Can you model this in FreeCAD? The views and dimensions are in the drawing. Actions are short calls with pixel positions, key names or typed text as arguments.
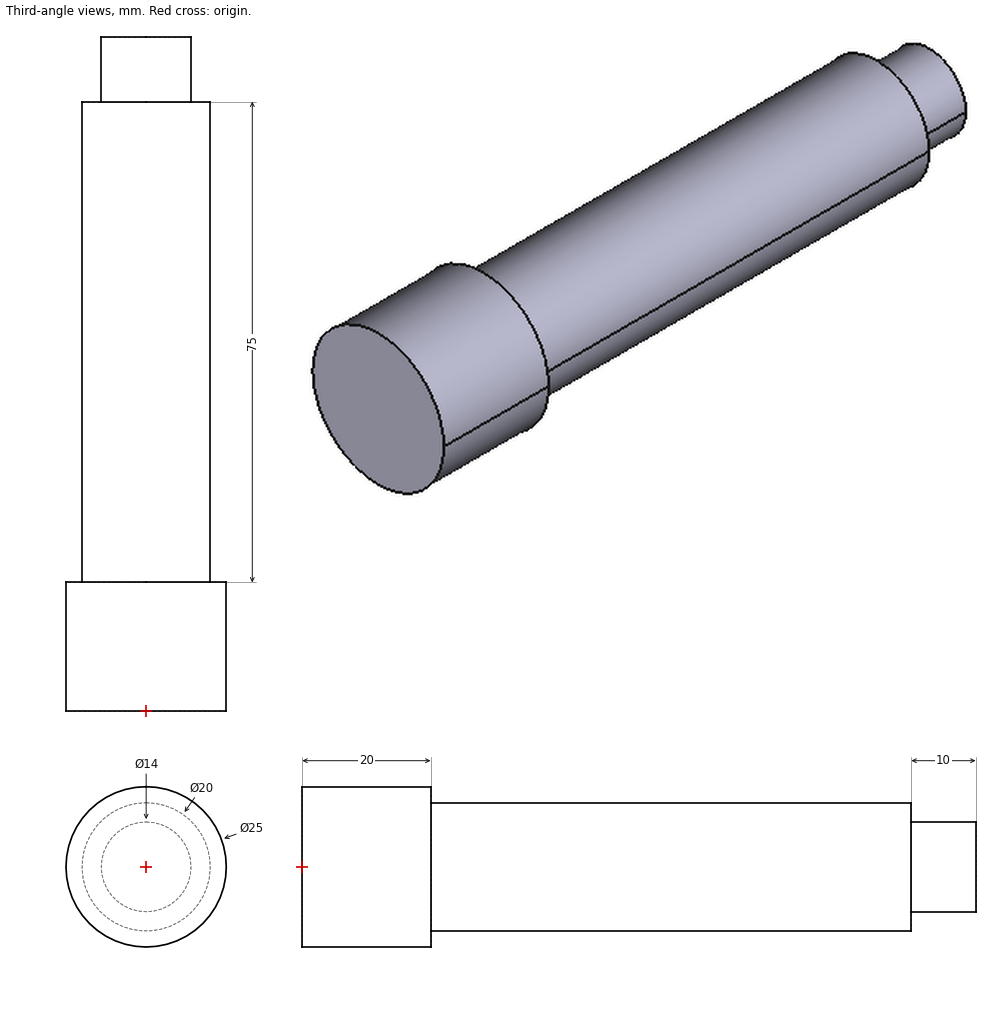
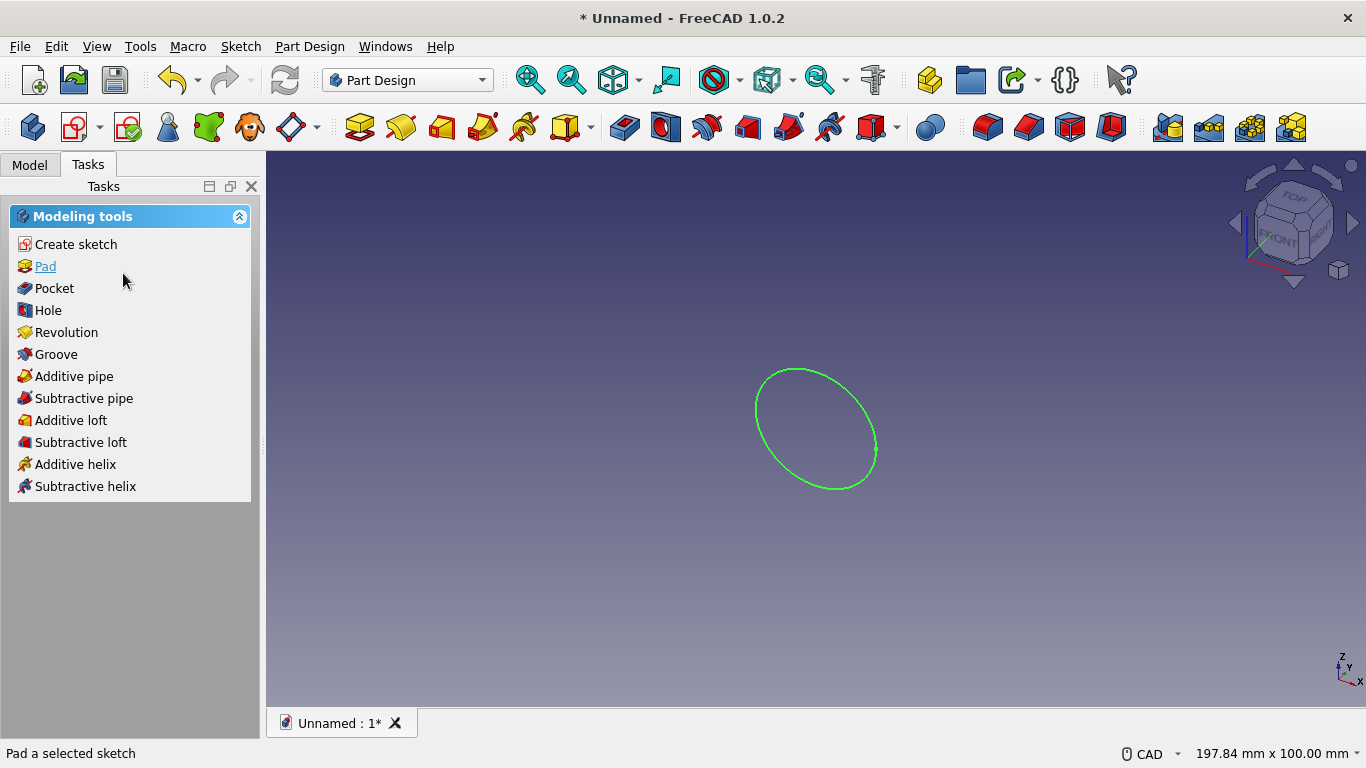
click(360, 128)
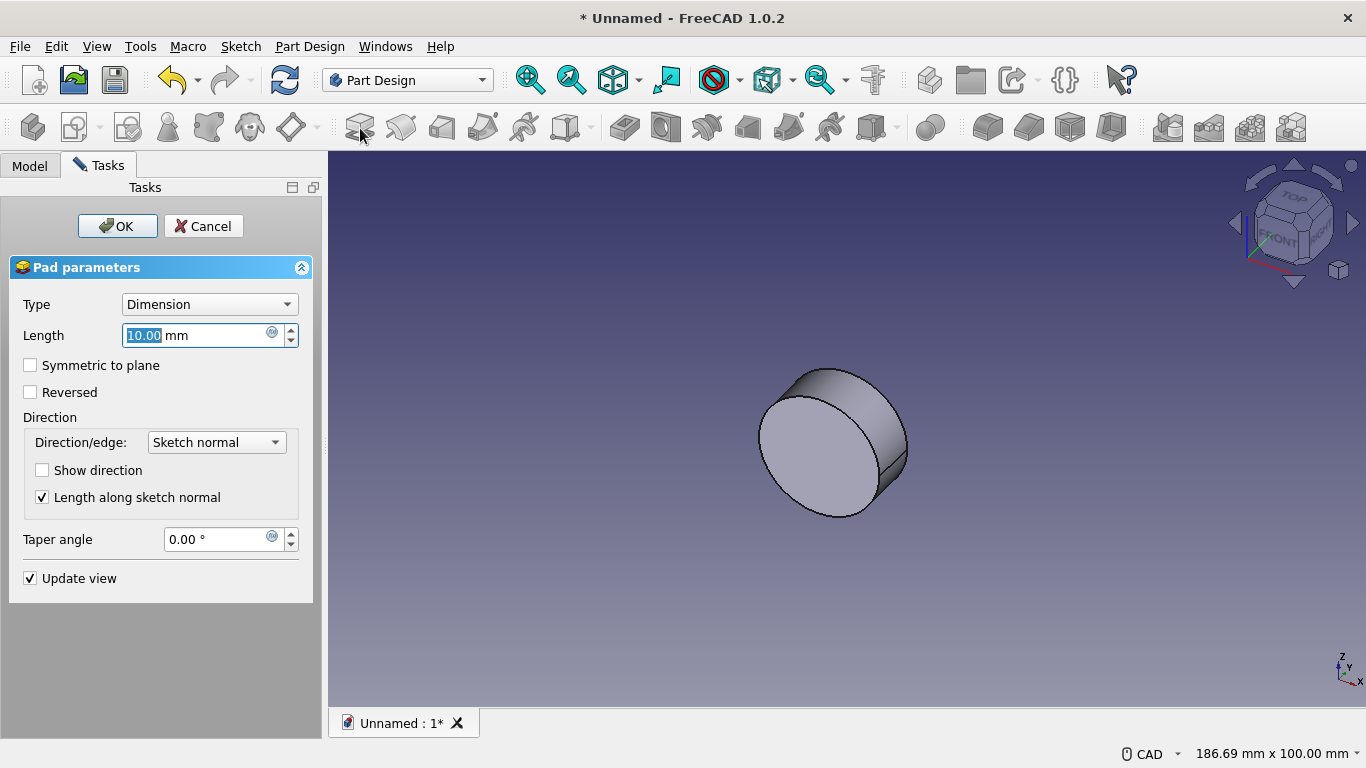
text(20)
key(Tab)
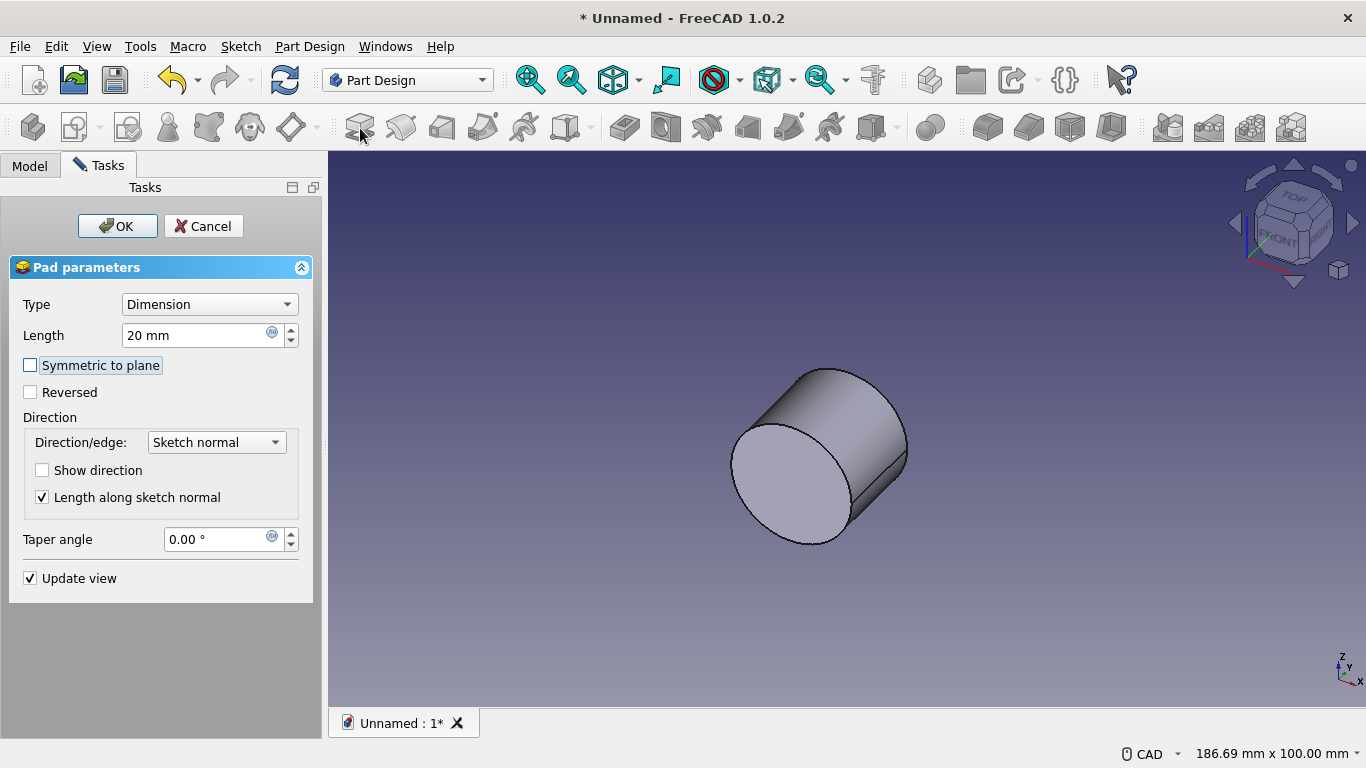
click(31, 392)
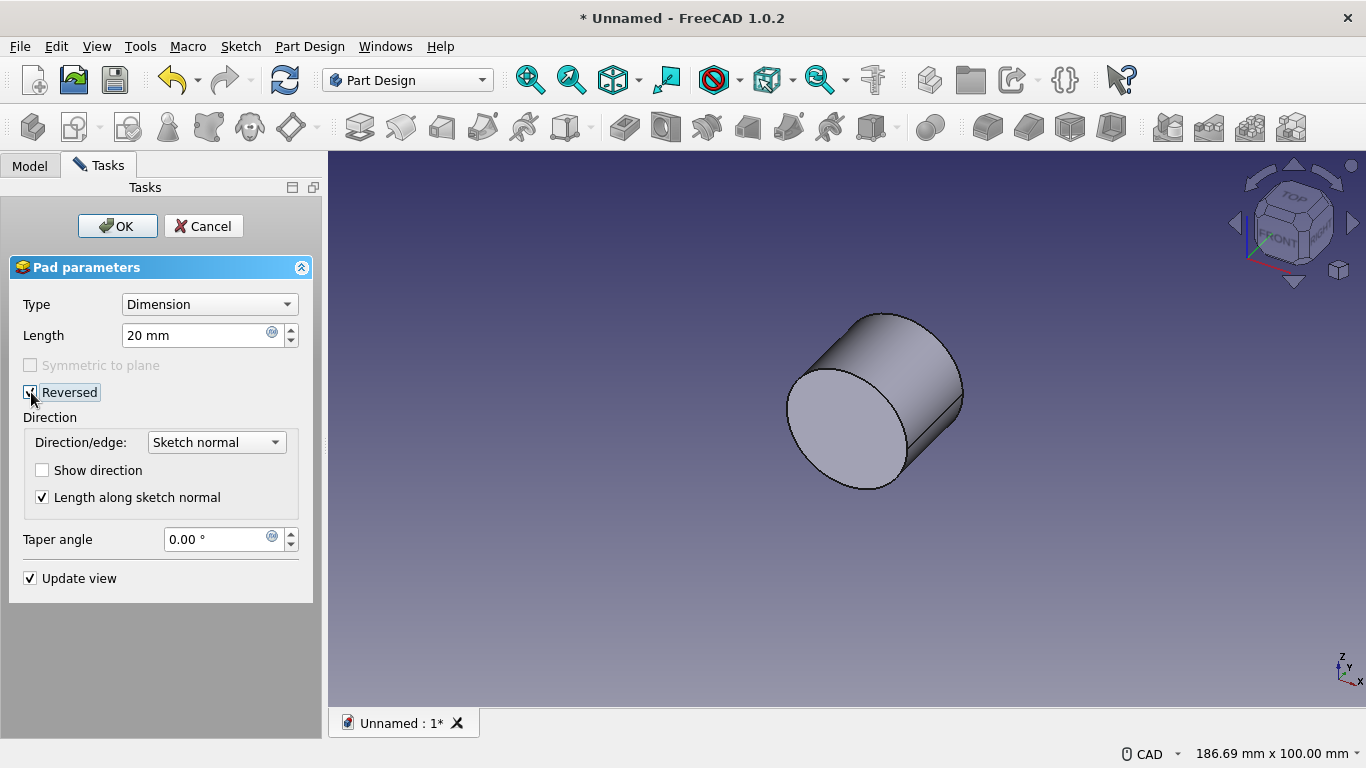
click(118, 226)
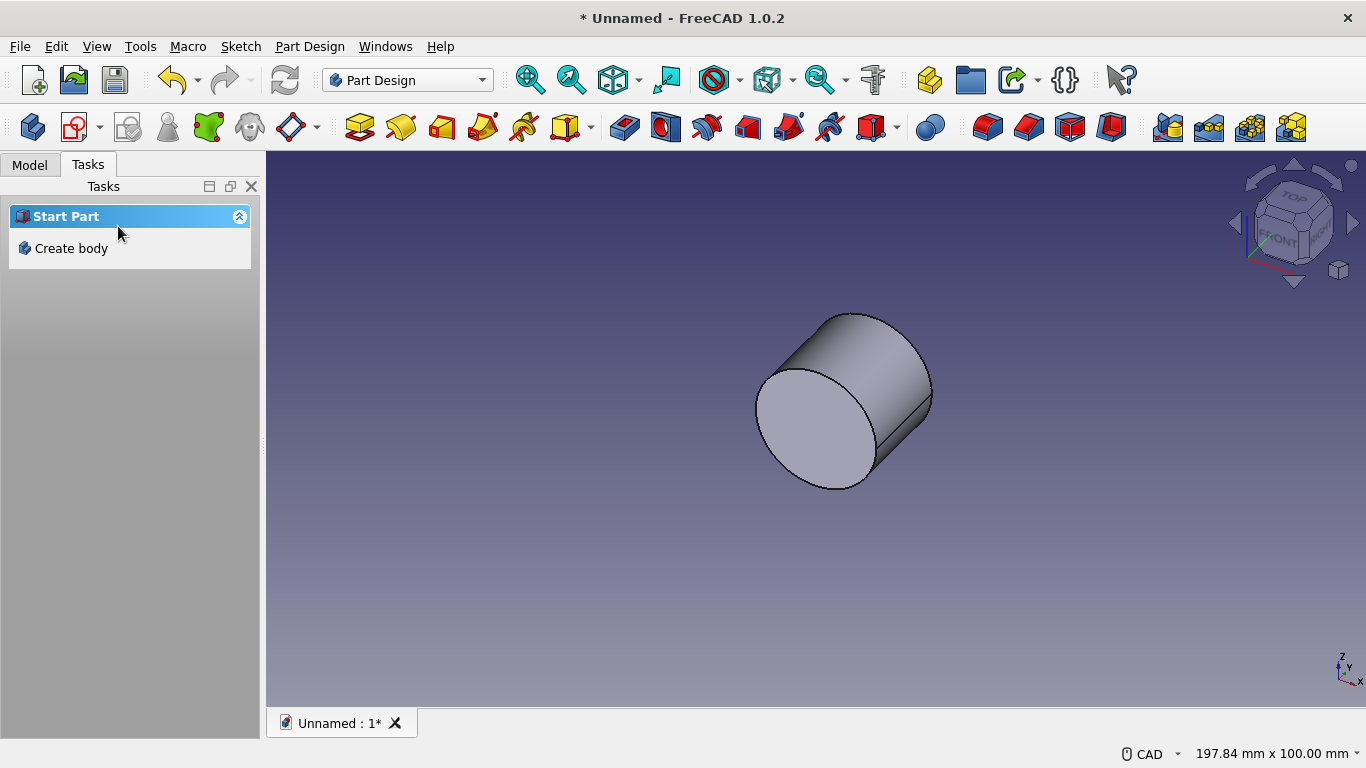
click(531, 80)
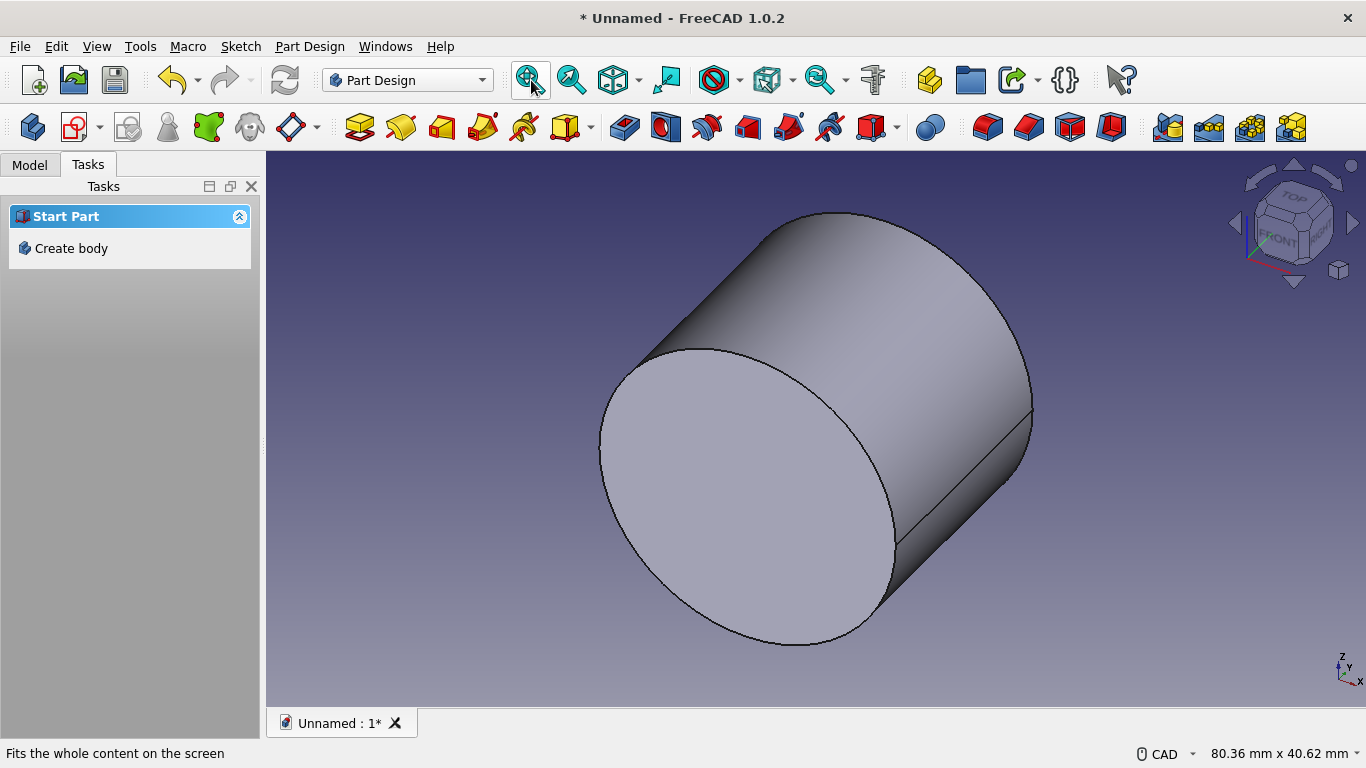
key(4)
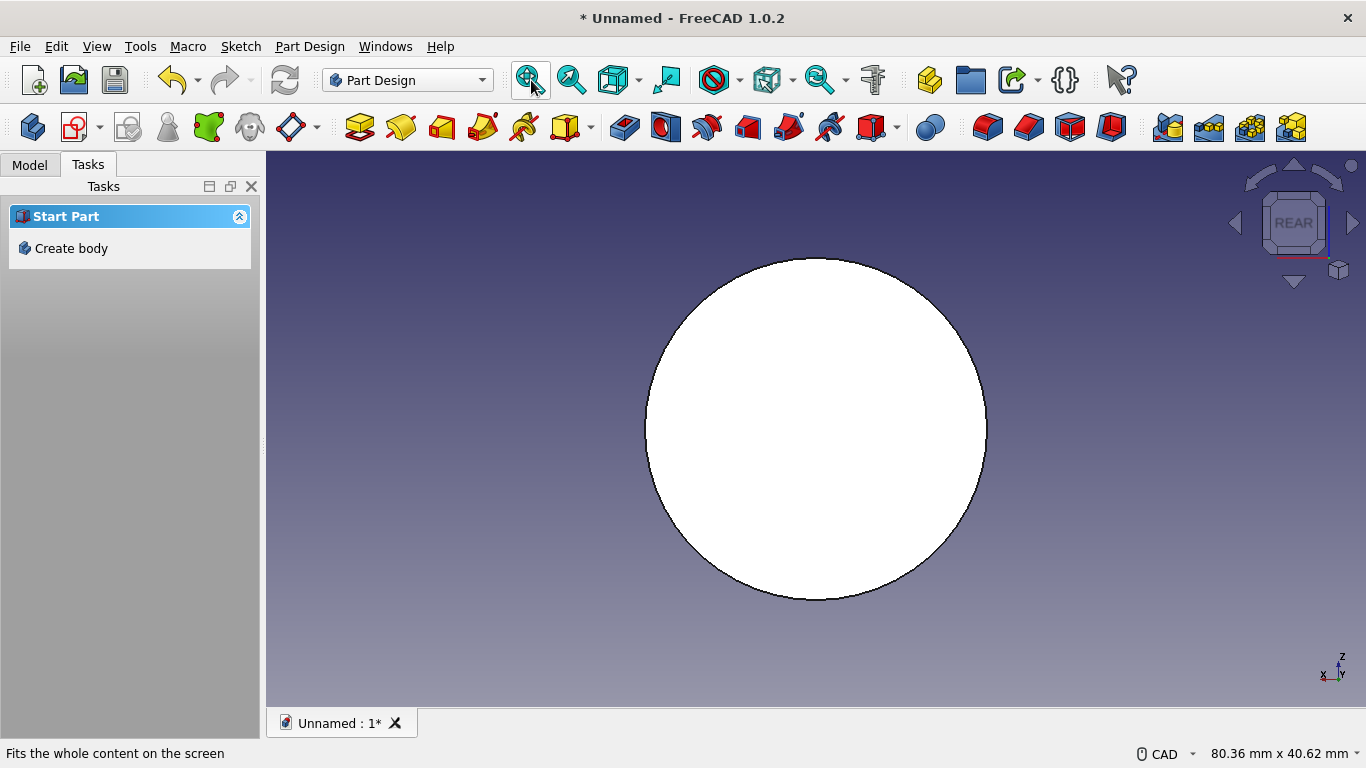
click(816, 428)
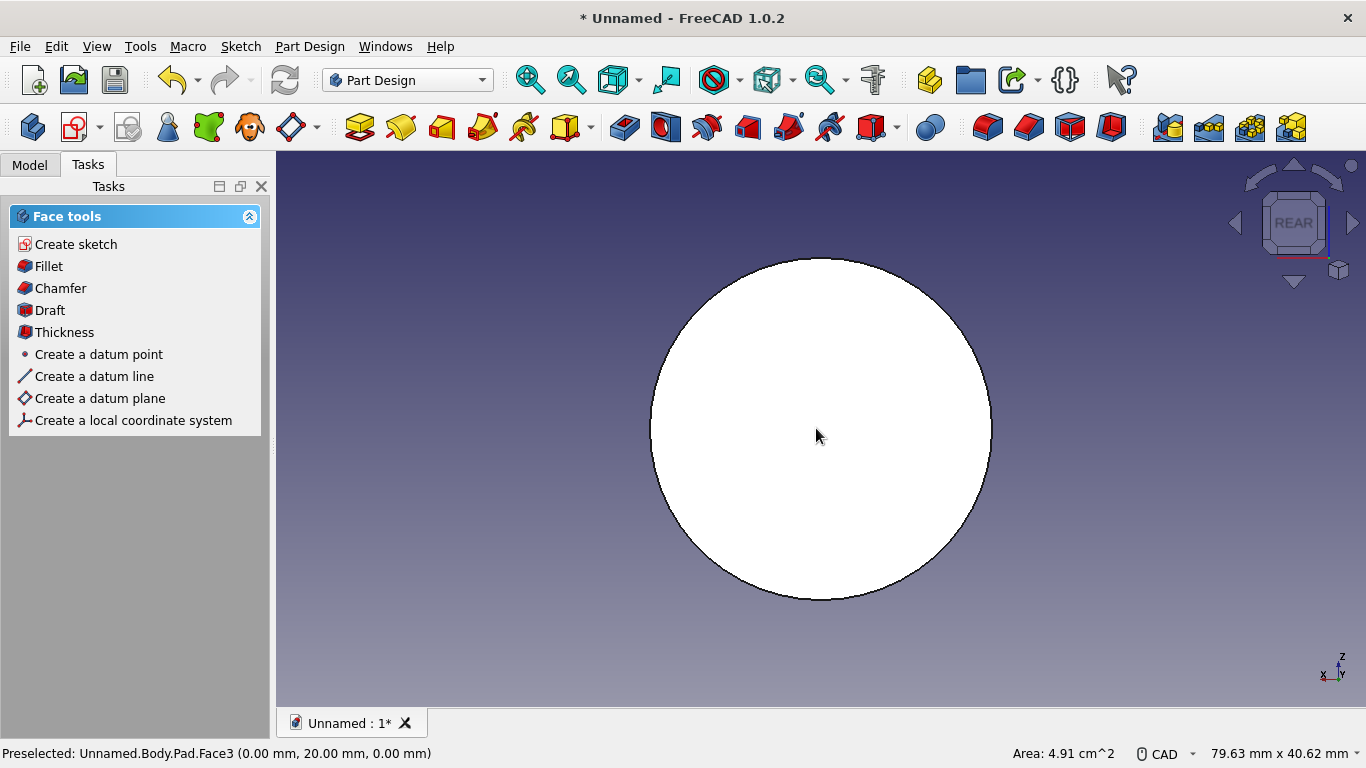
click(74, 128)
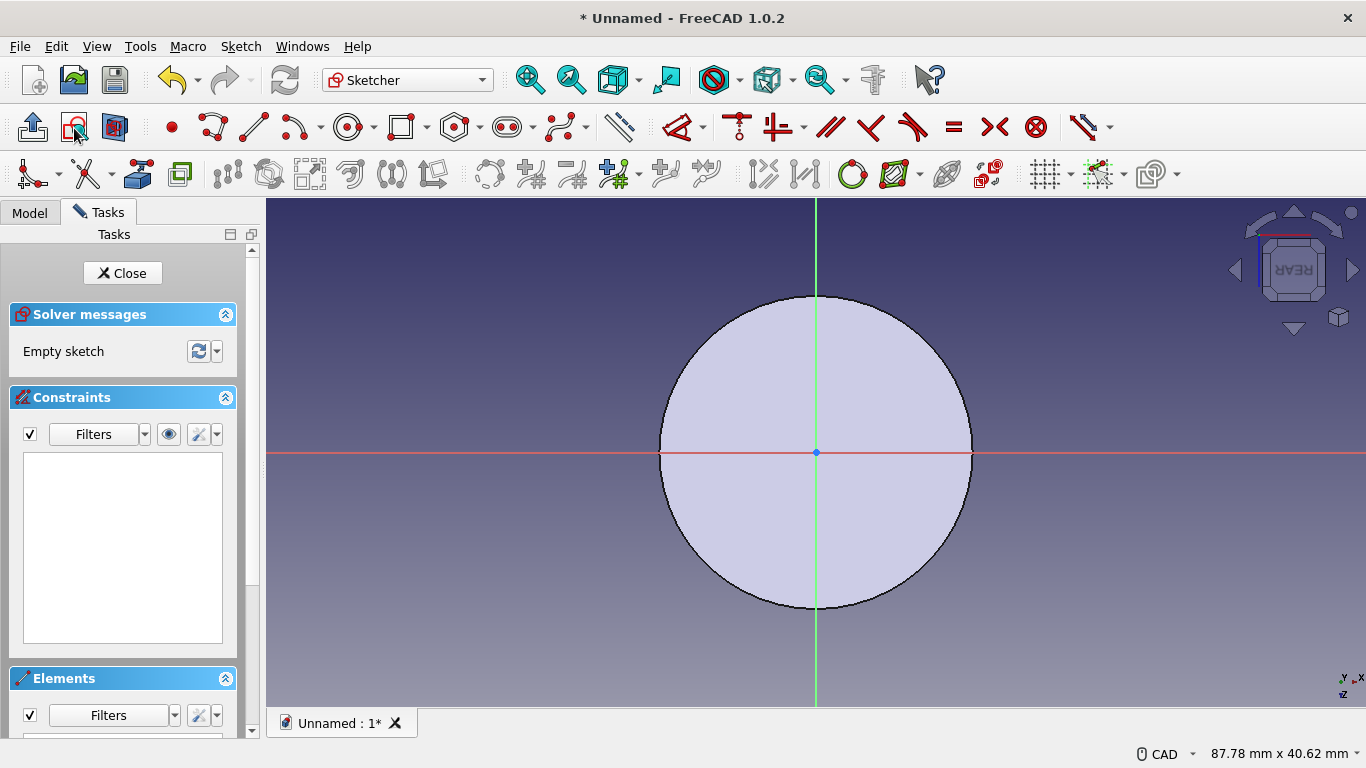
click(348, 128)